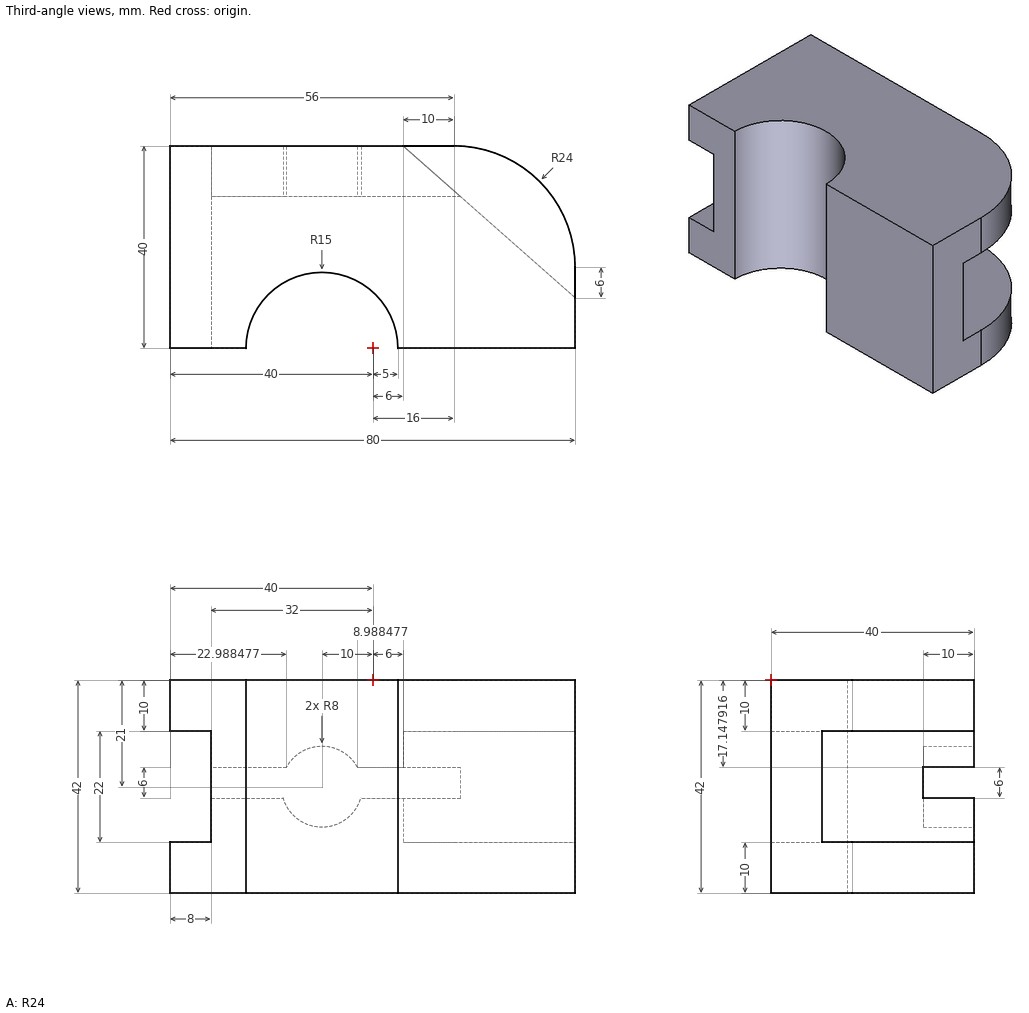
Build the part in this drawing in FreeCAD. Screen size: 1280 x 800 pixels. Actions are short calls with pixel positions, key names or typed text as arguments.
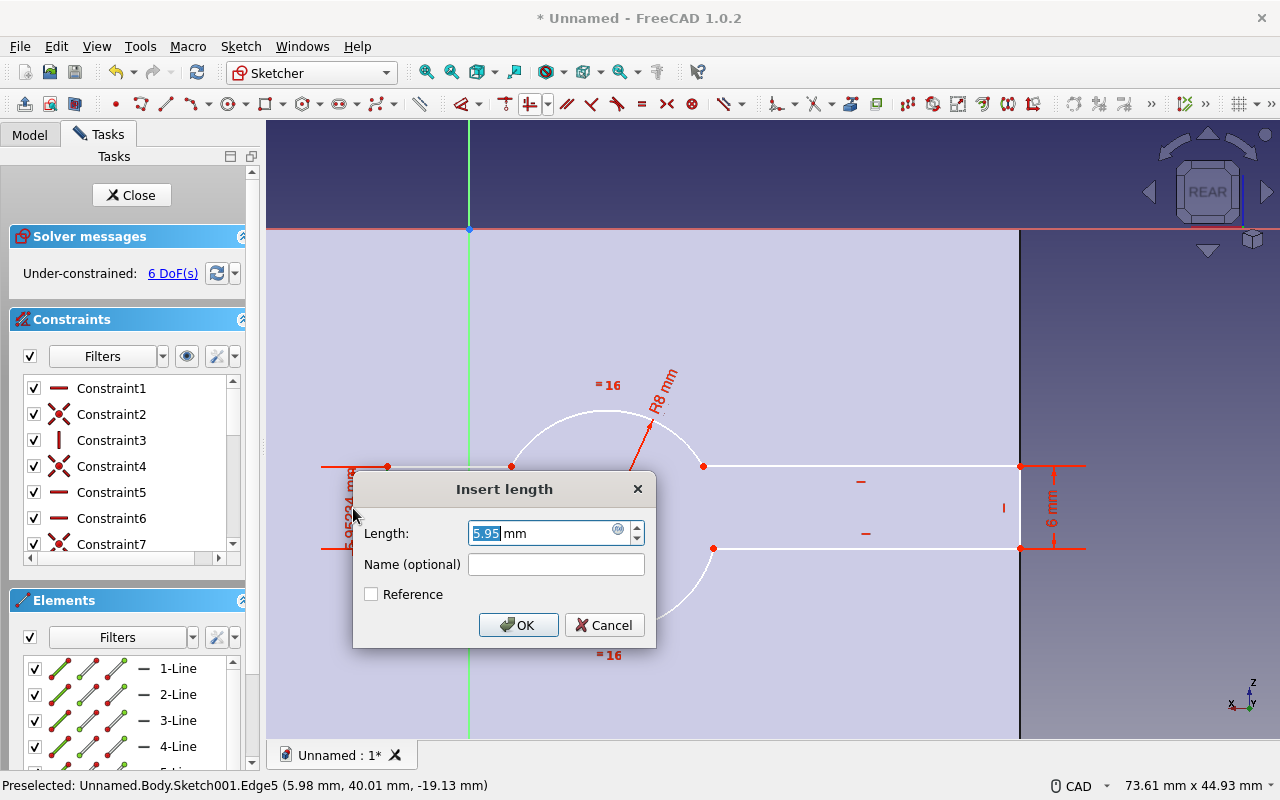
text(6)
key(Return)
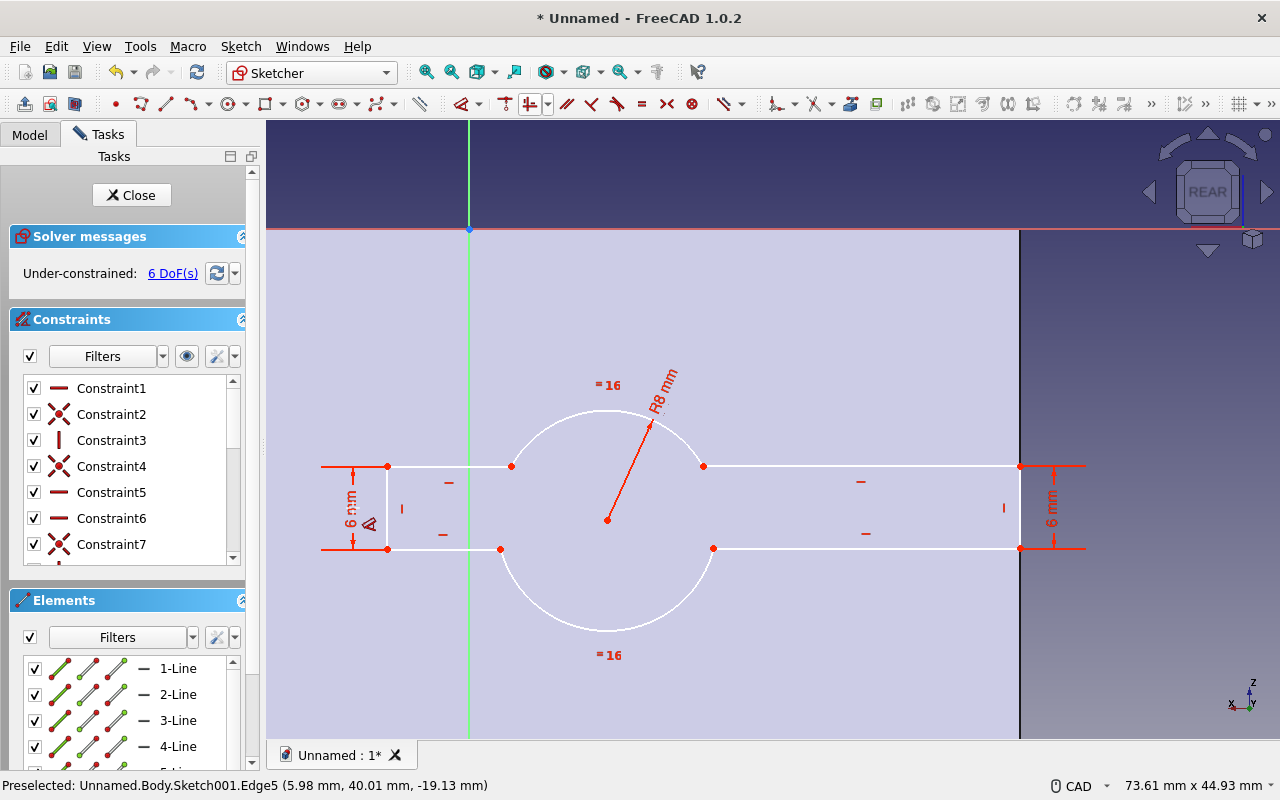
click(387, 467)
click(428, 195)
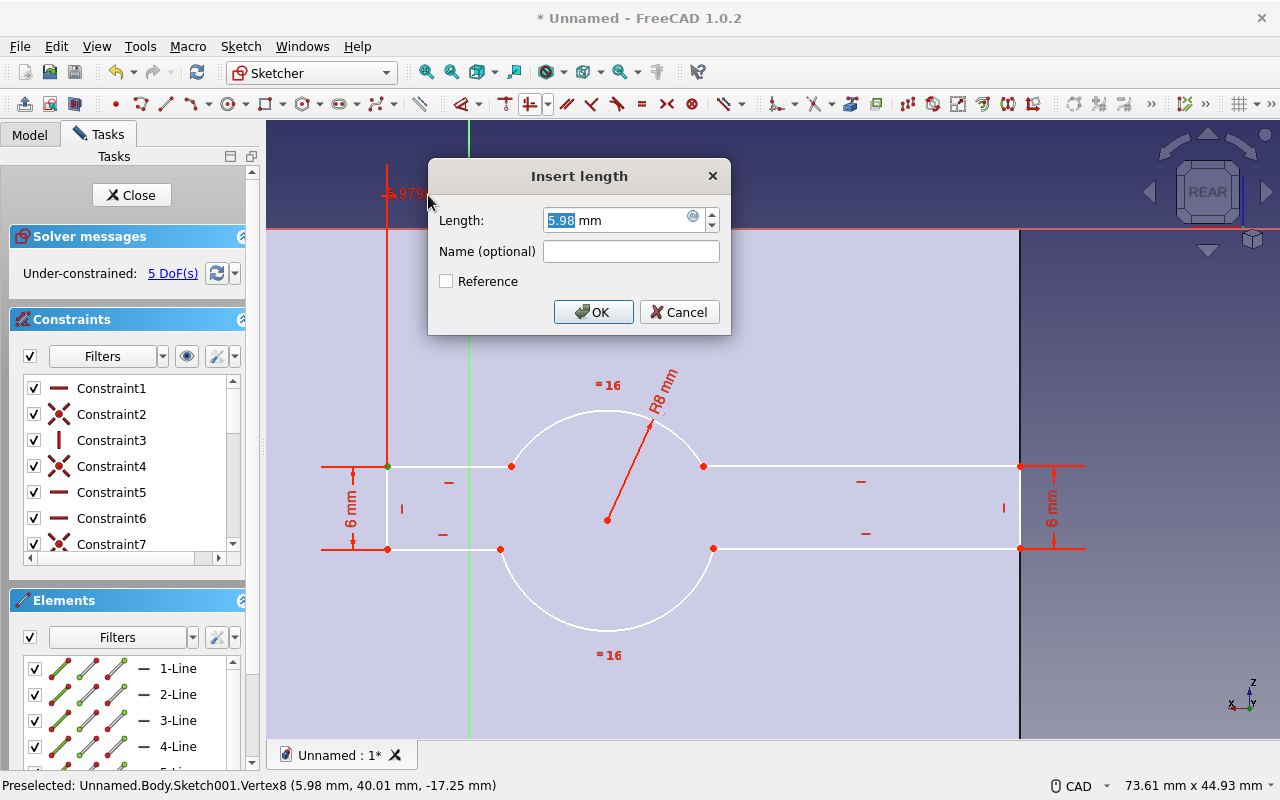
text(6)
key(Return)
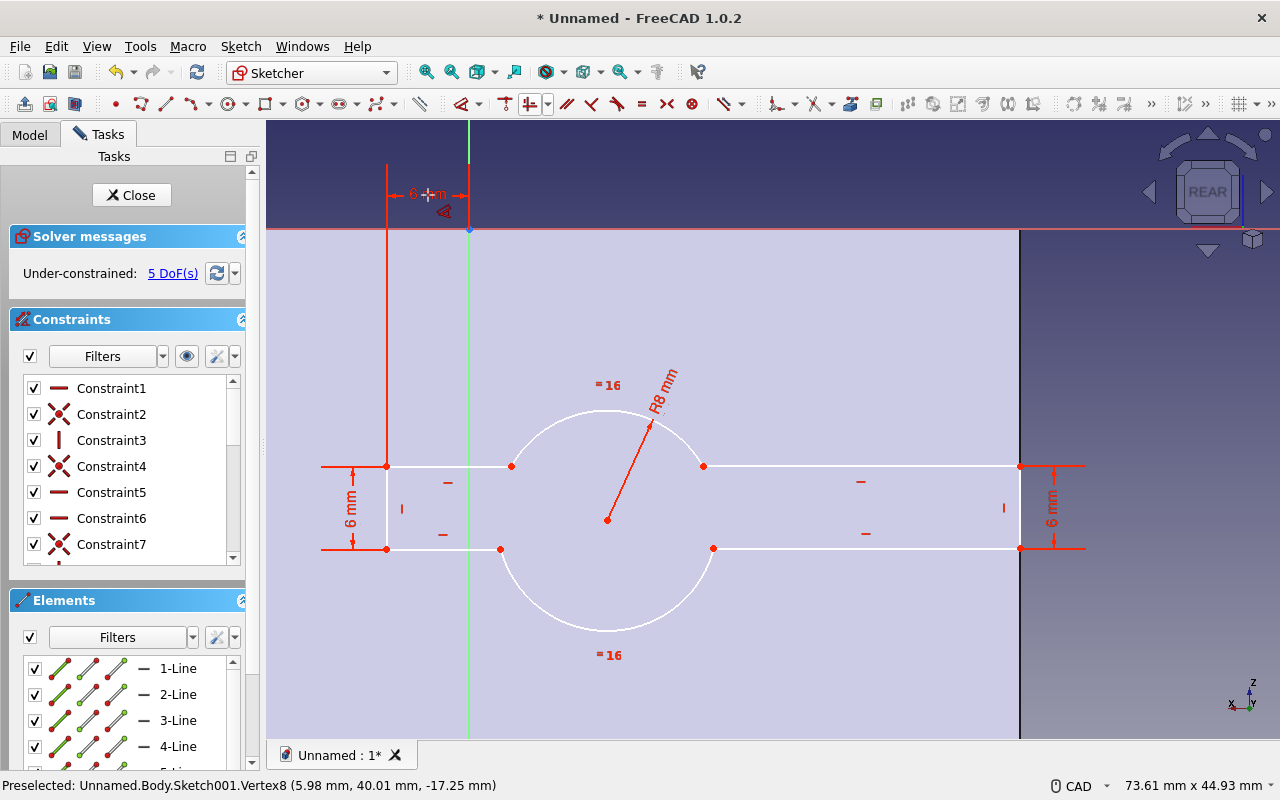
click(1020, 549)
click(745, 195)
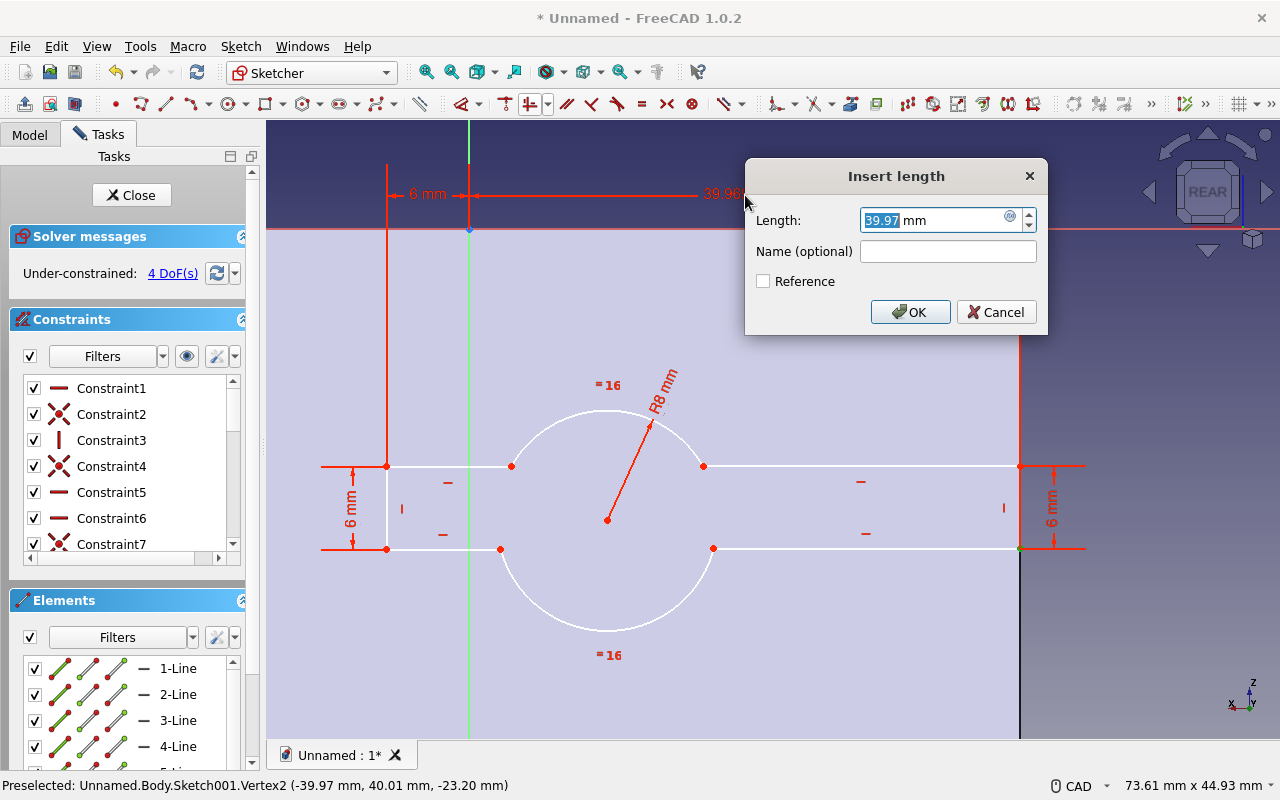
text(40)
key(Return)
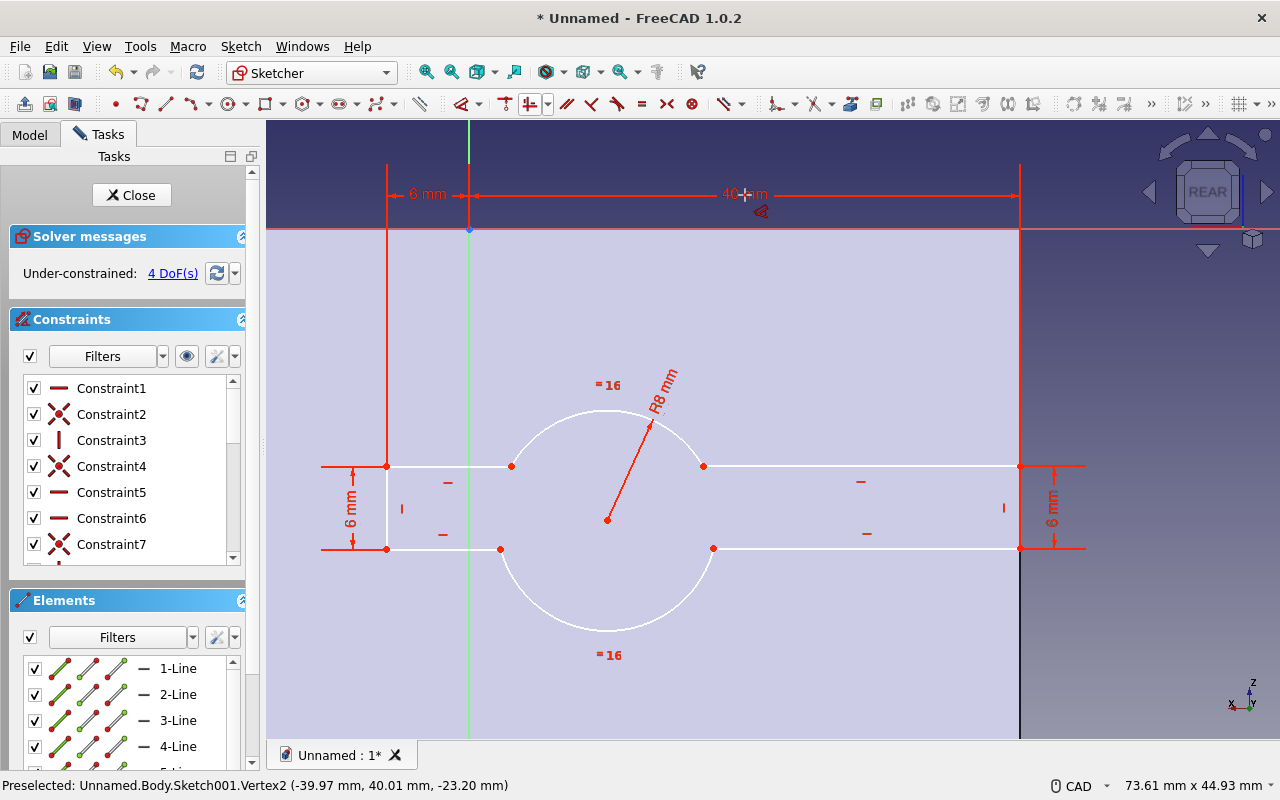
click(607, 521)
click(538, 195)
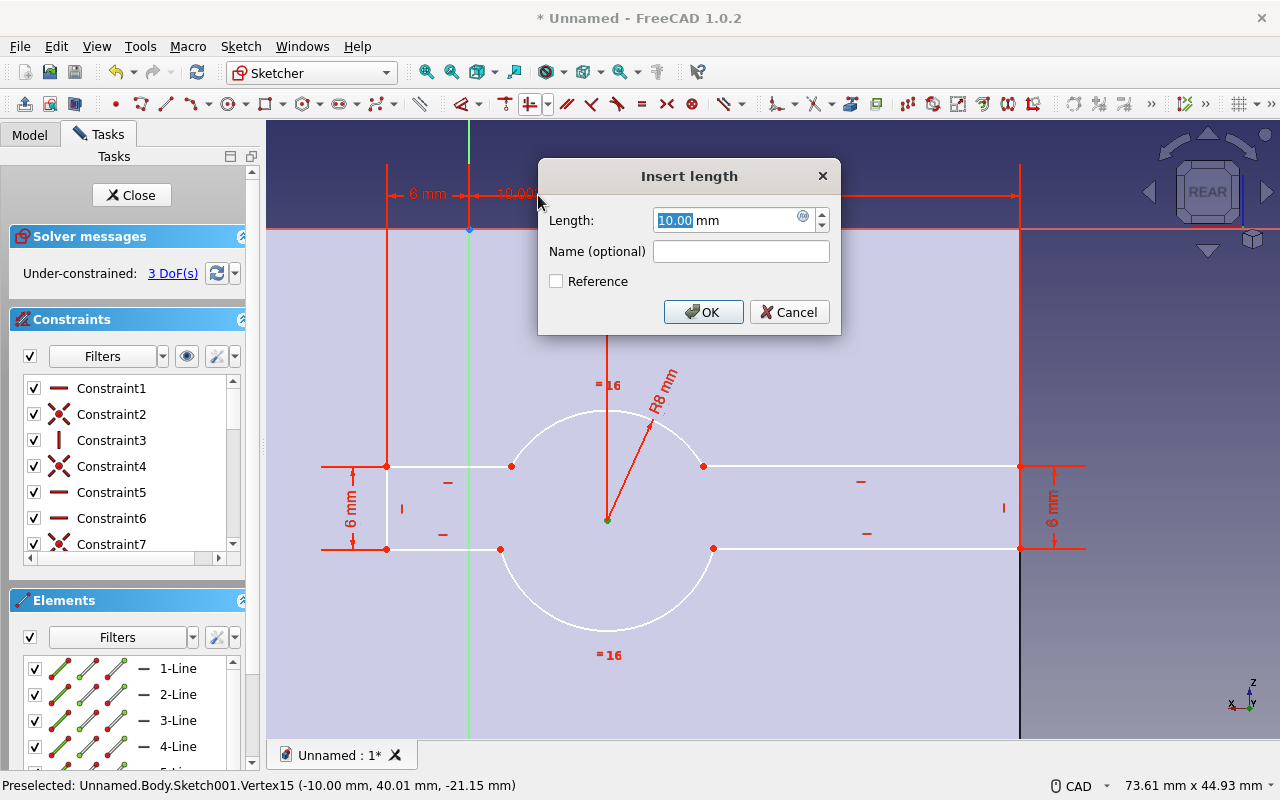
text(10)
key(Return)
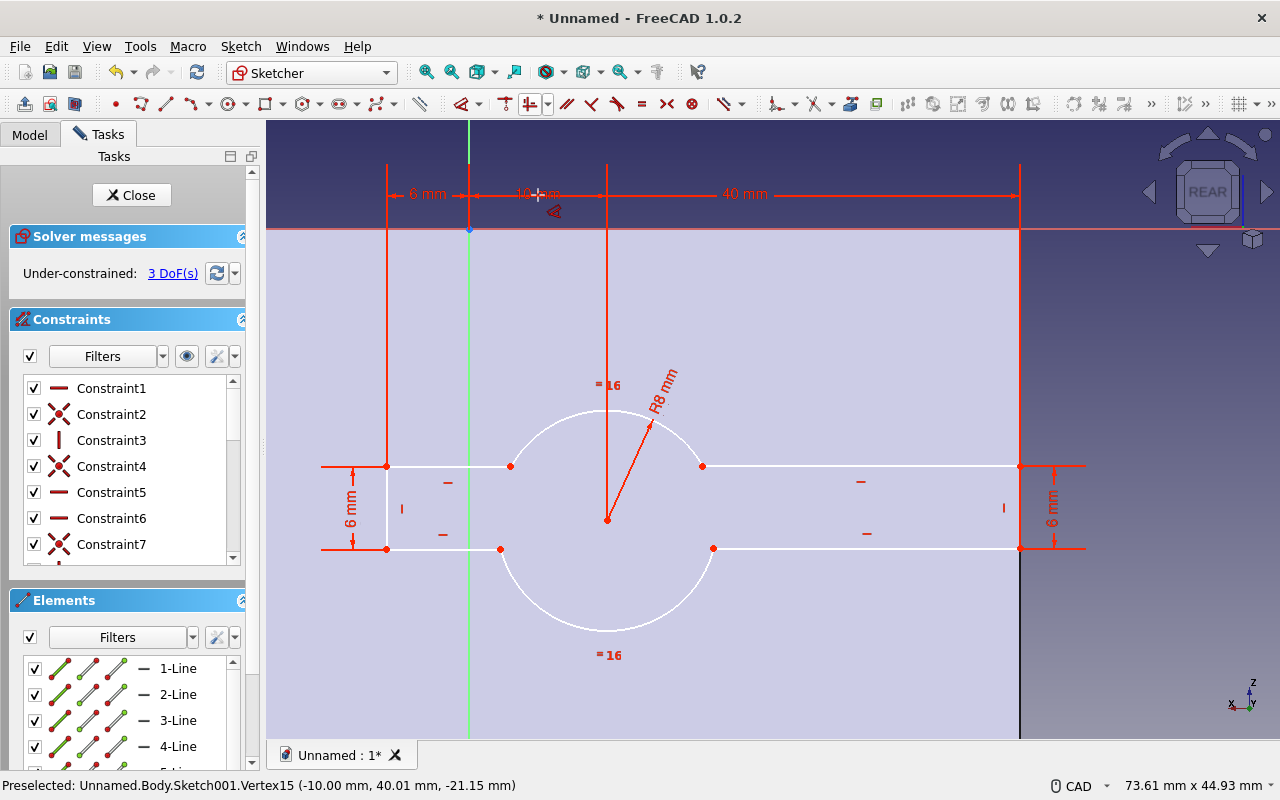
click(607, 521)
click(435, 375)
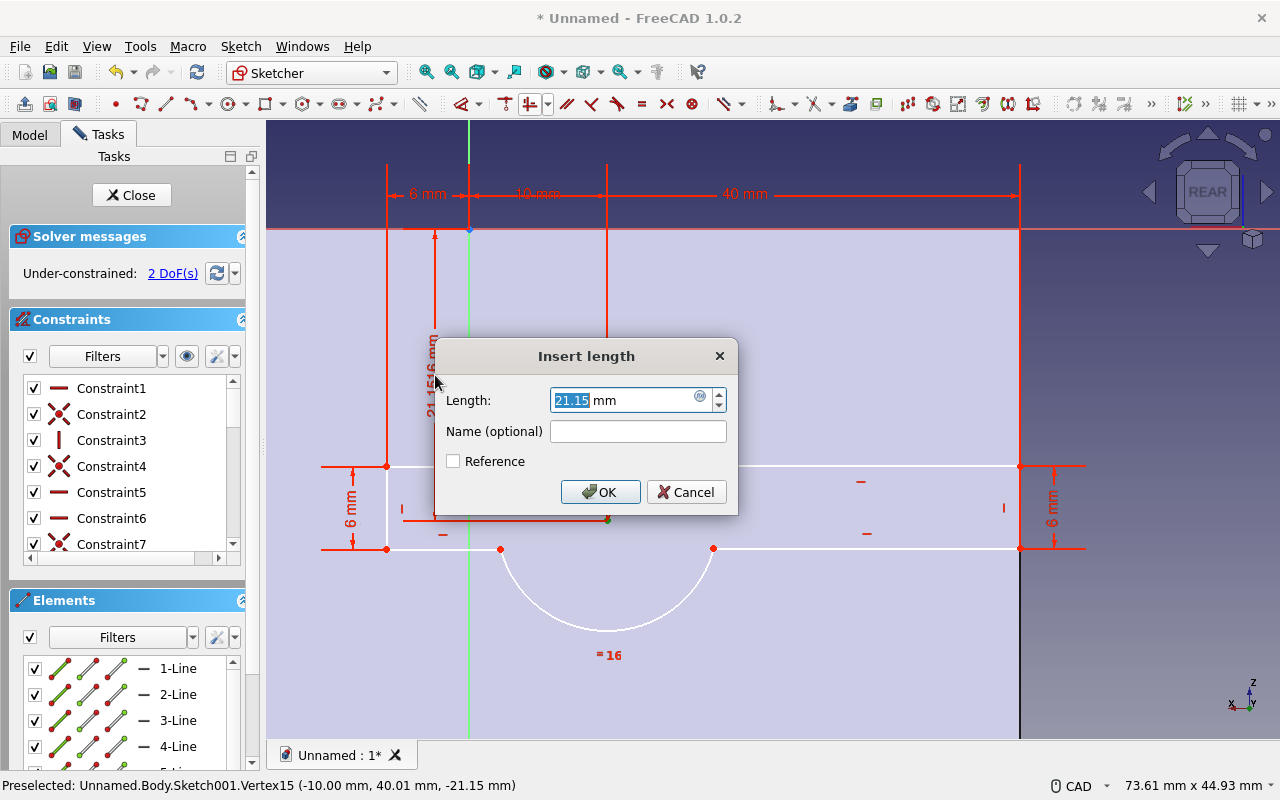
text(21)
key(Return)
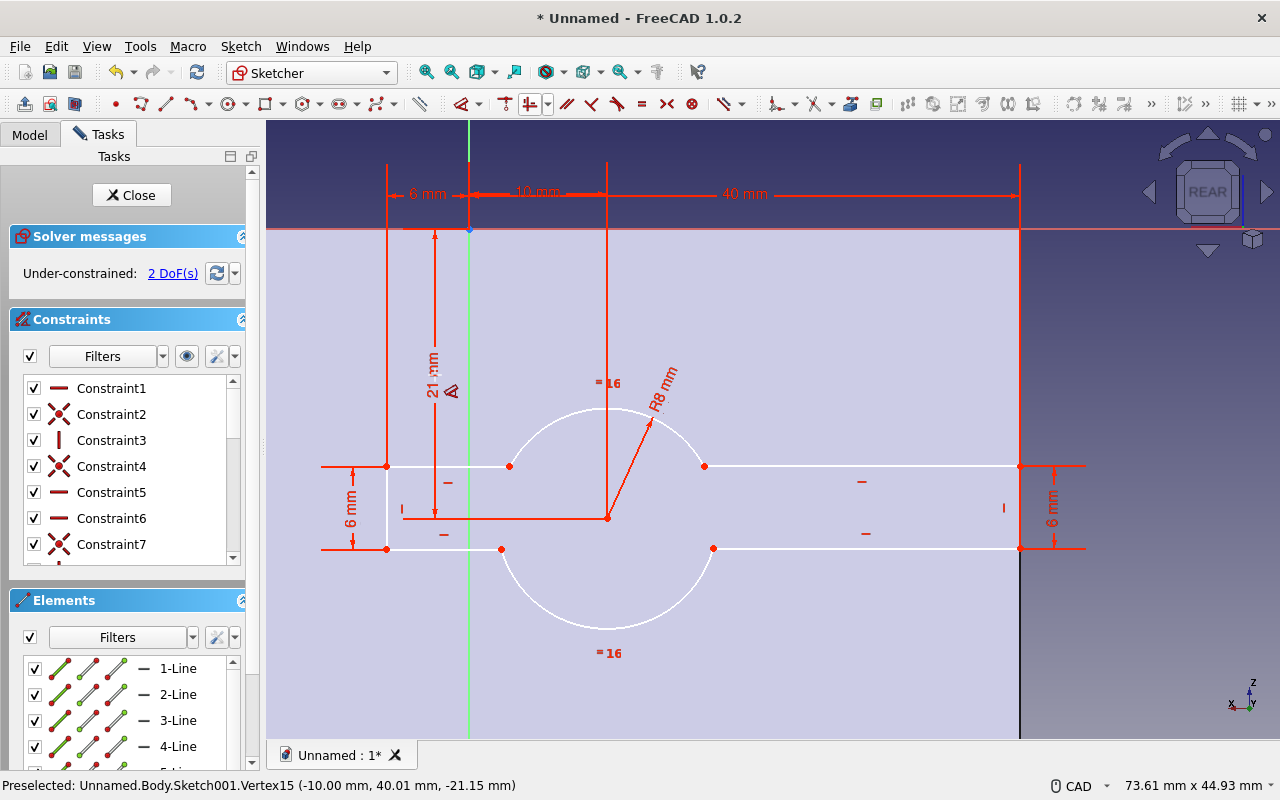
click(473, 467)
click(448, 501)